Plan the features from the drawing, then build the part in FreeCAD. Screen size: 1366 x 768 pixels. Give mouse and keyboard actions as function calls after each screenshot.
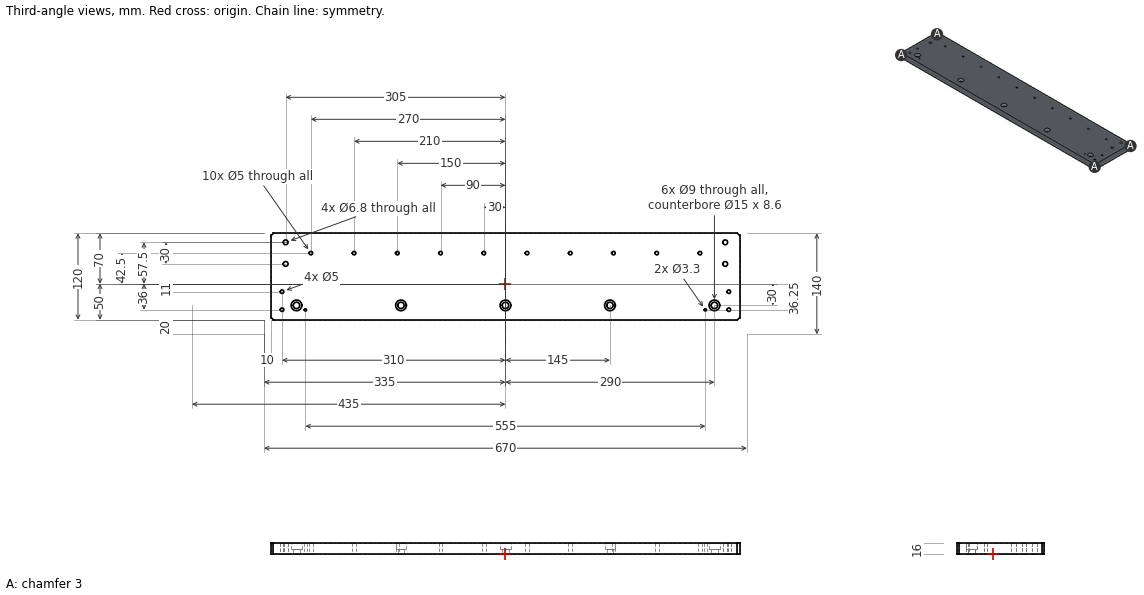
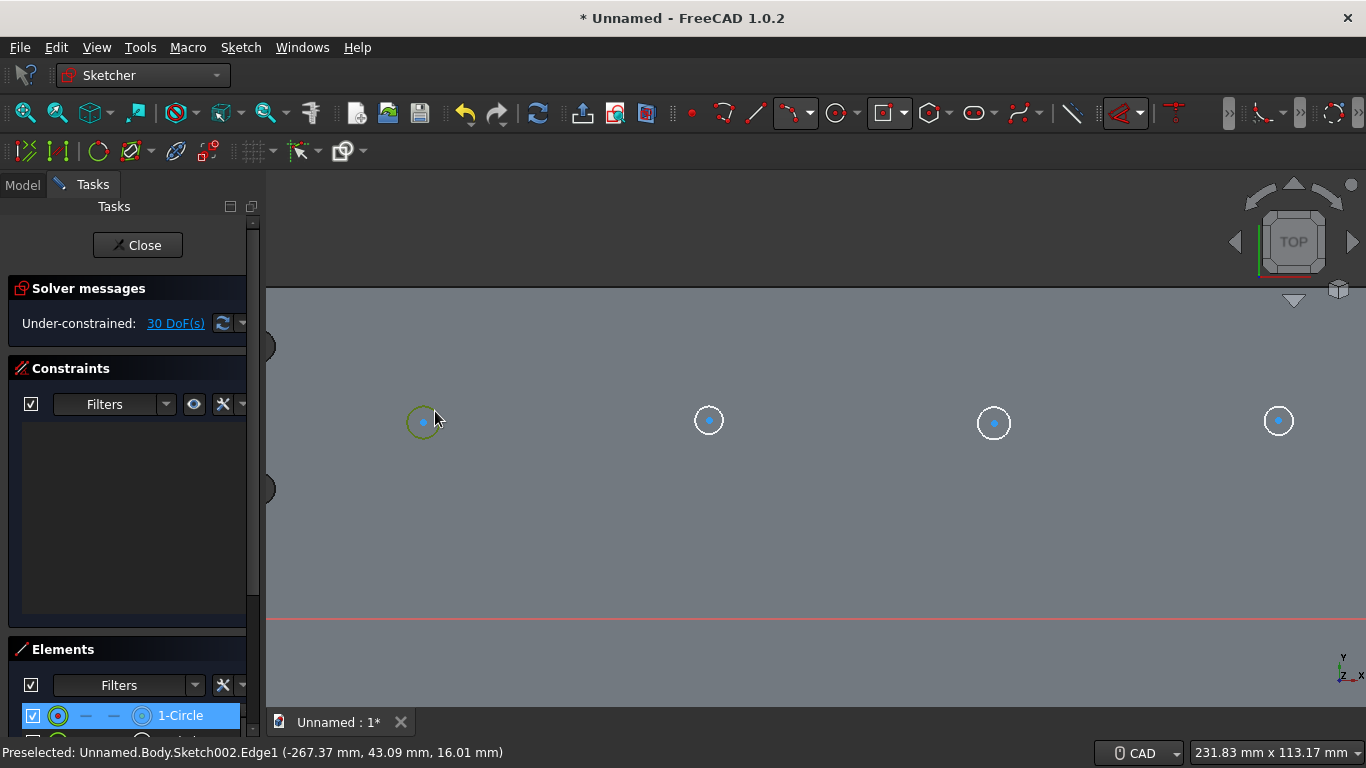
click(719, 410)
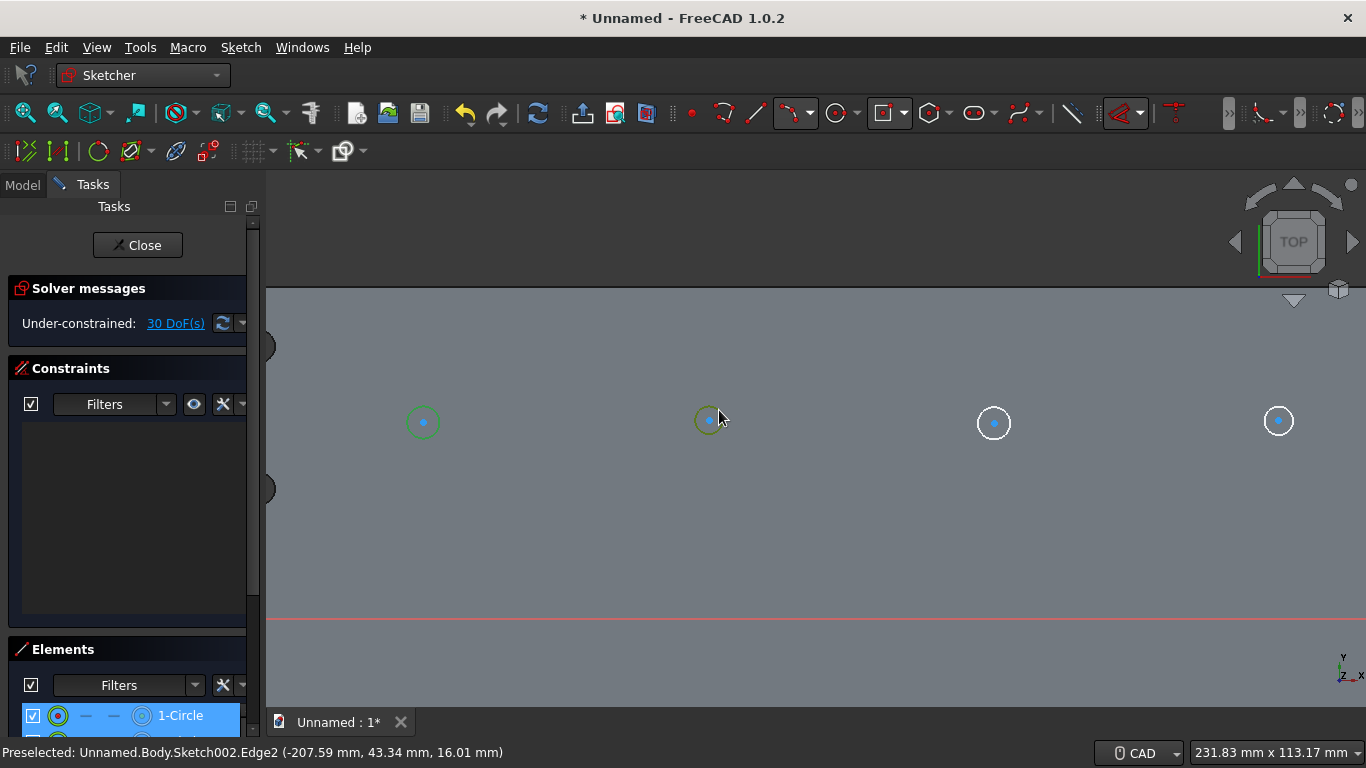
click(1005, 412)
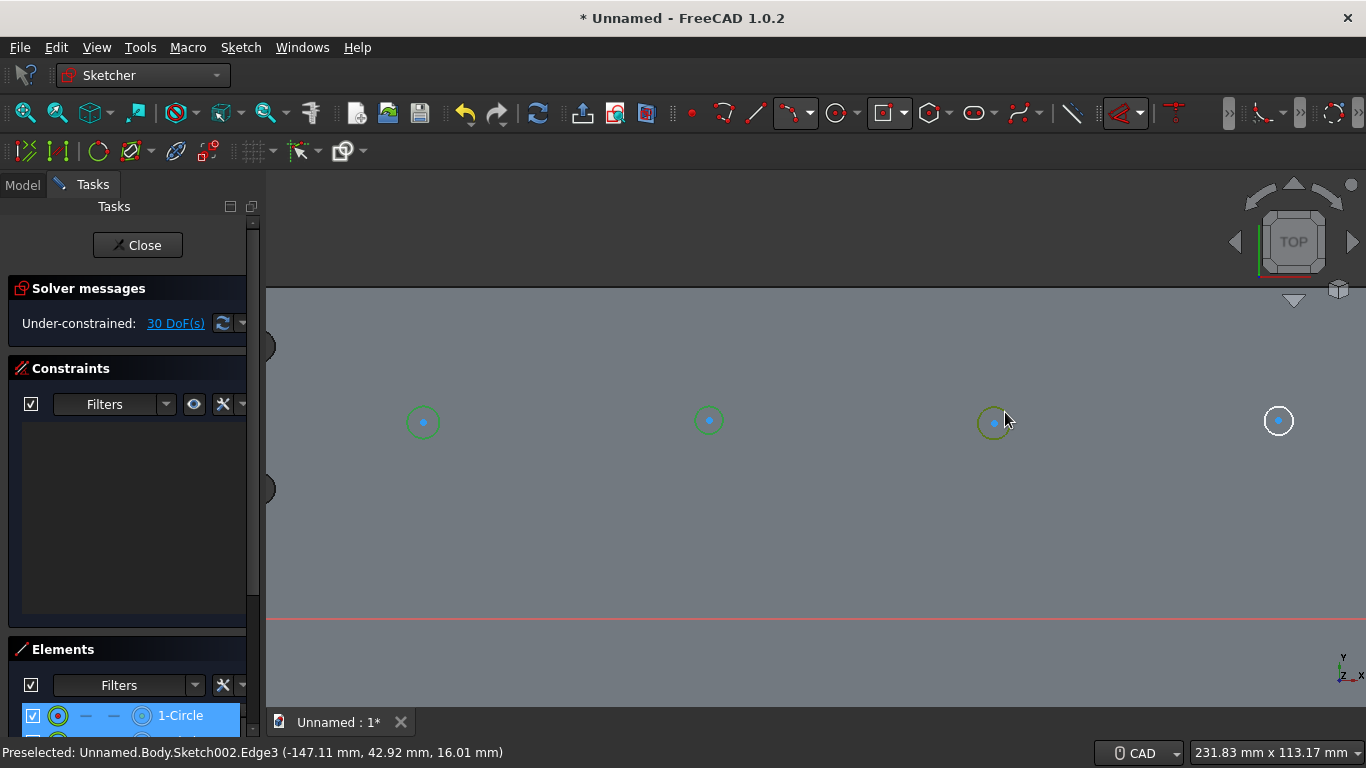
scroll(434, 414, down, 7)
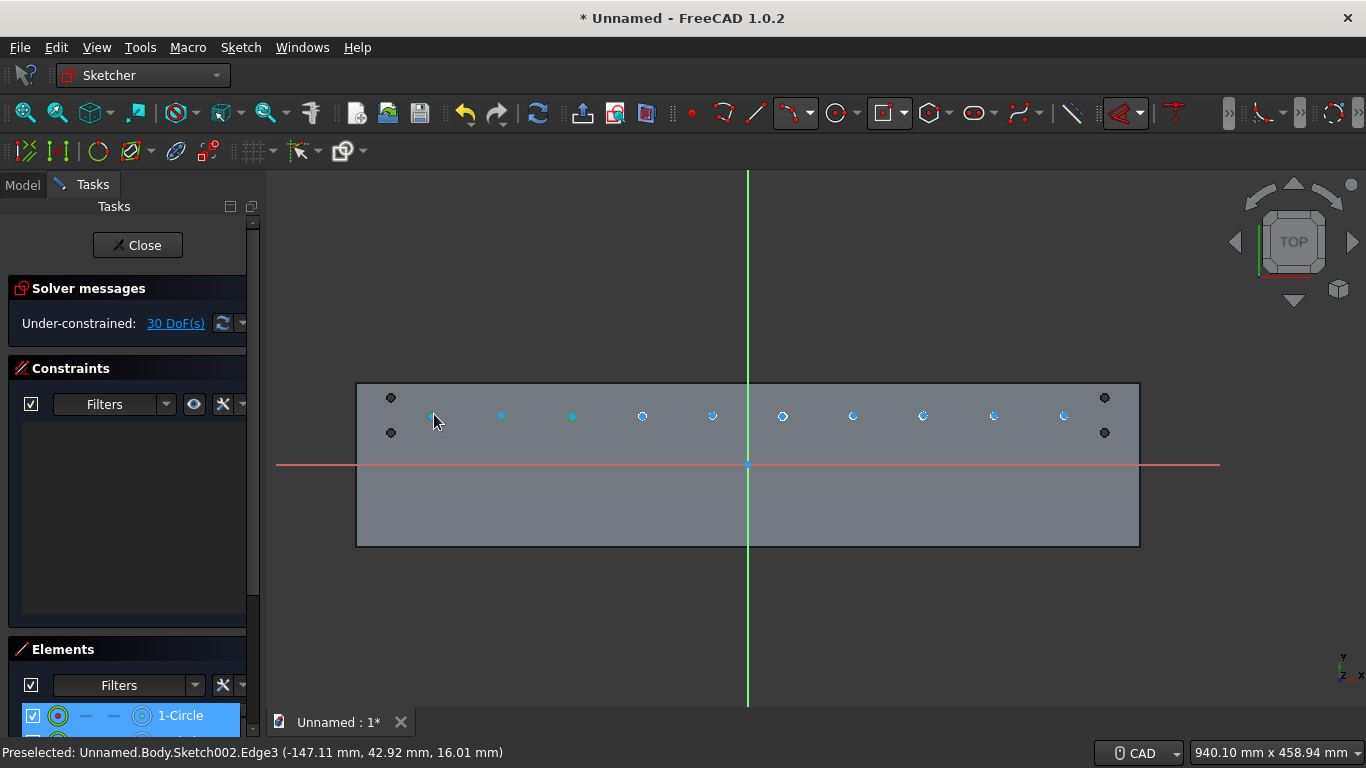
scroll(645, 414, up, 7)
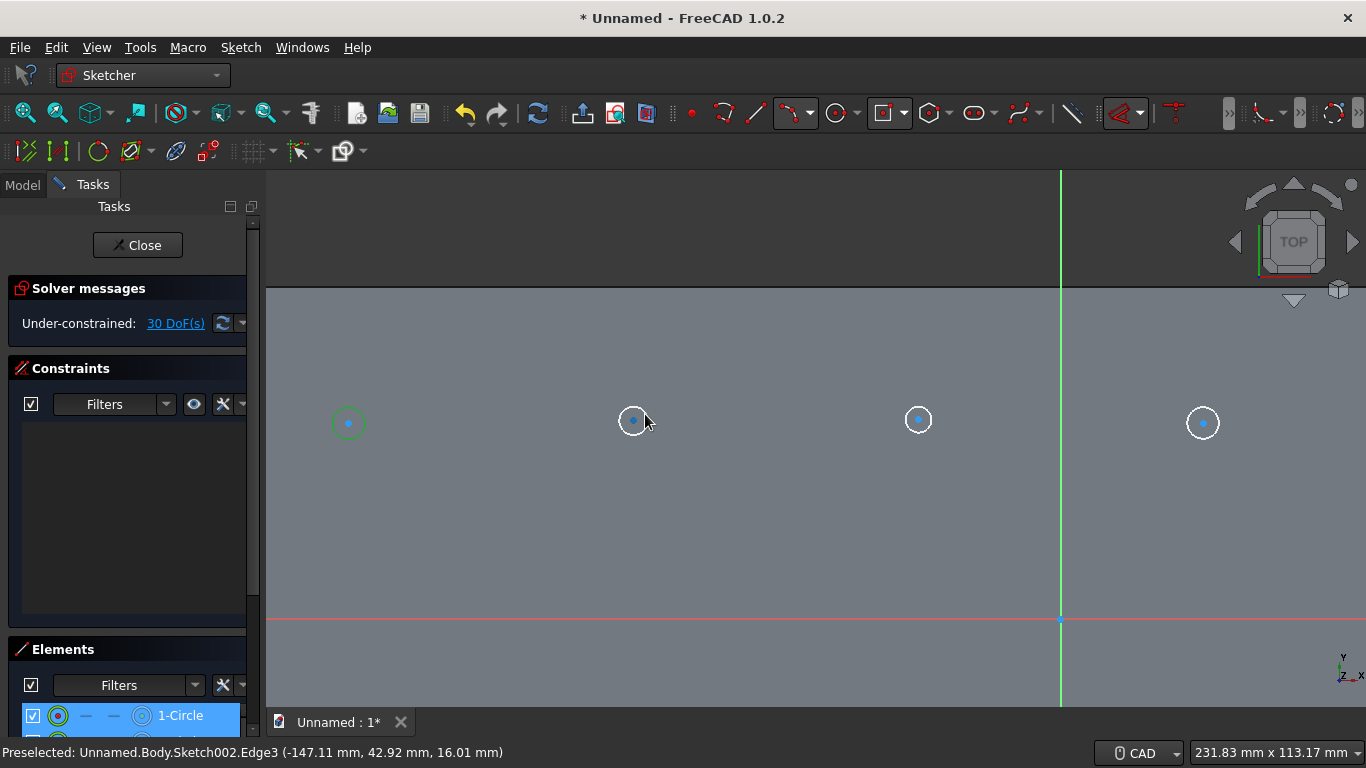
click(644, 411)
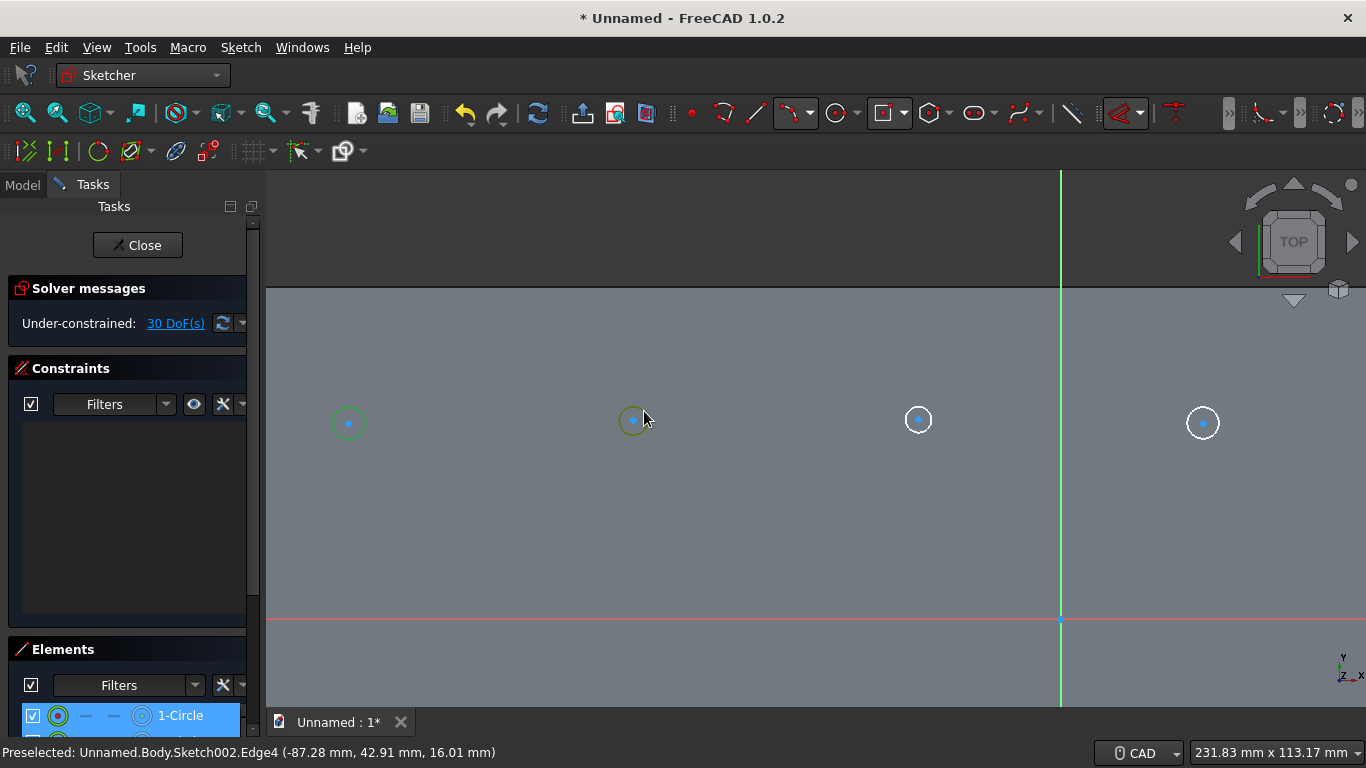
click(928, 411)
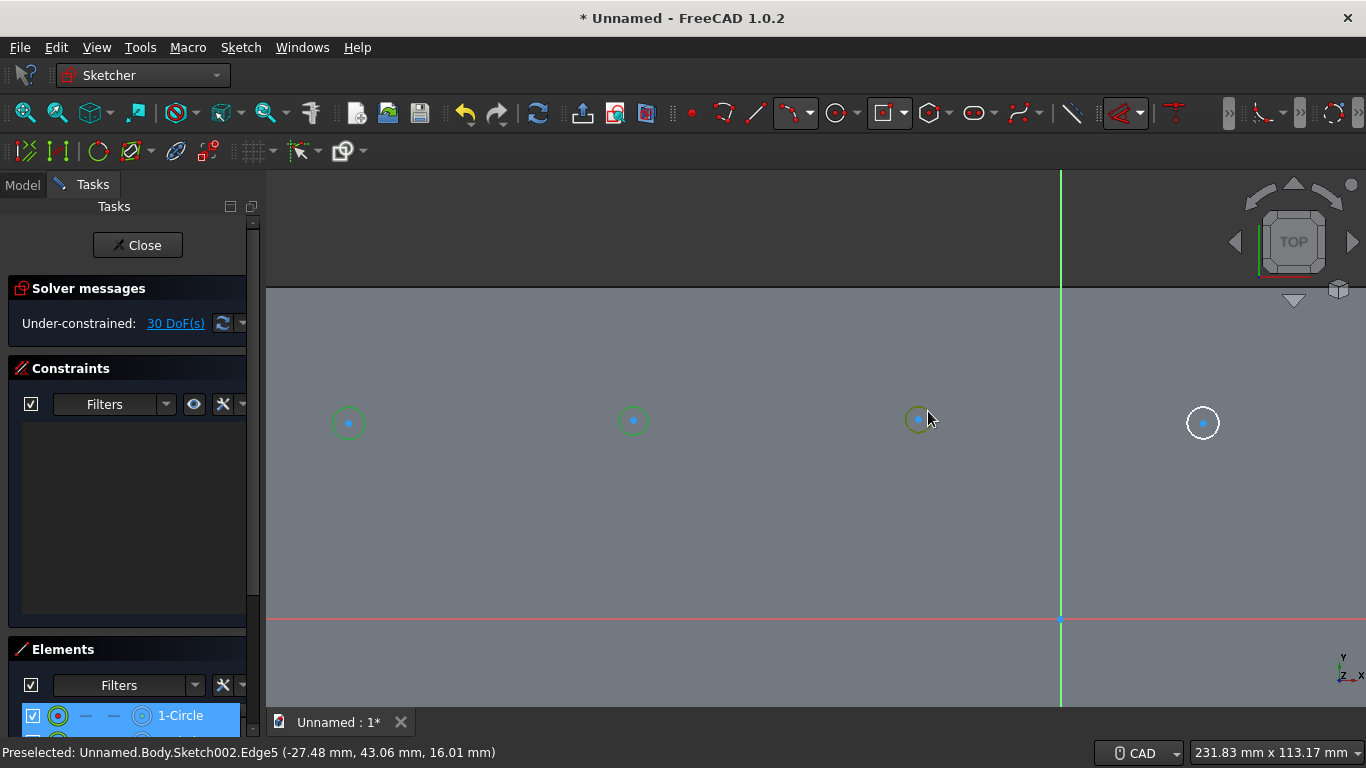
click(1192, 412)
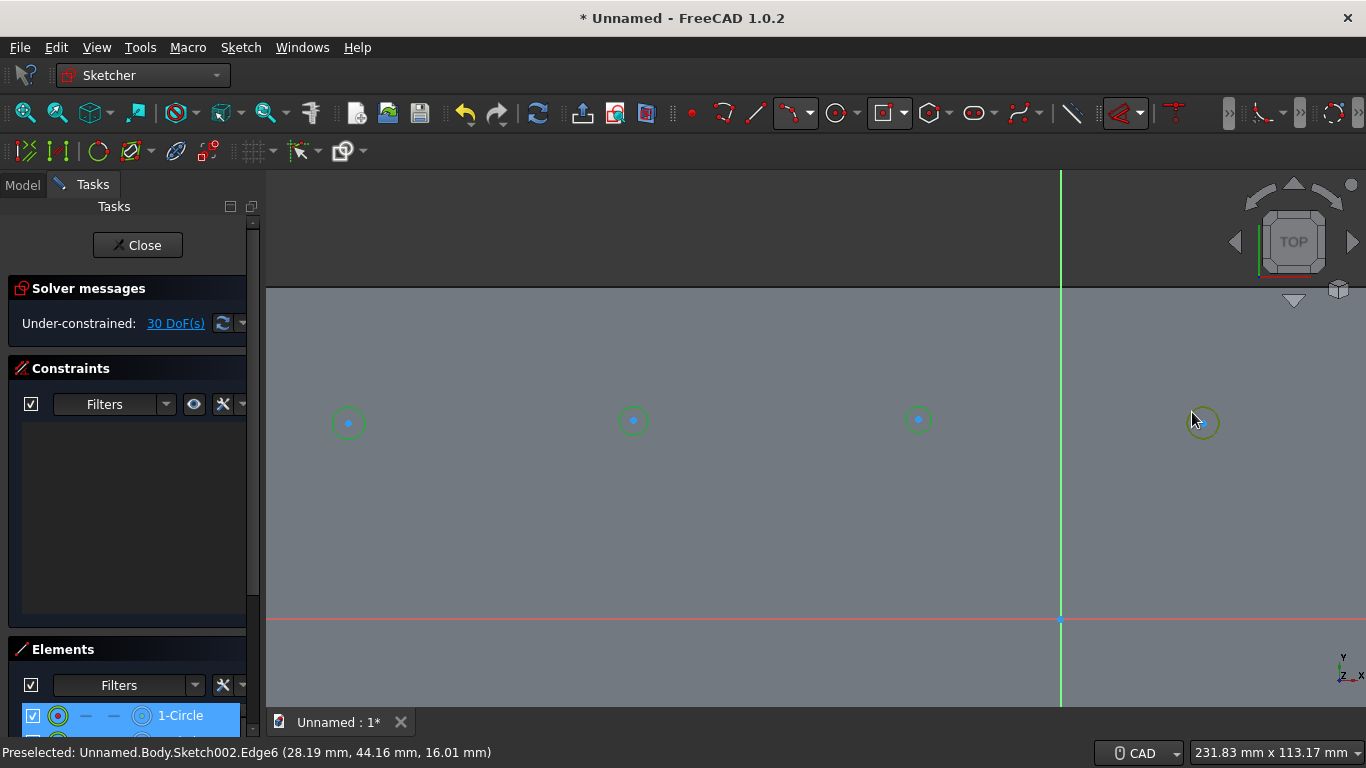
scroll(645, 414, down, 7)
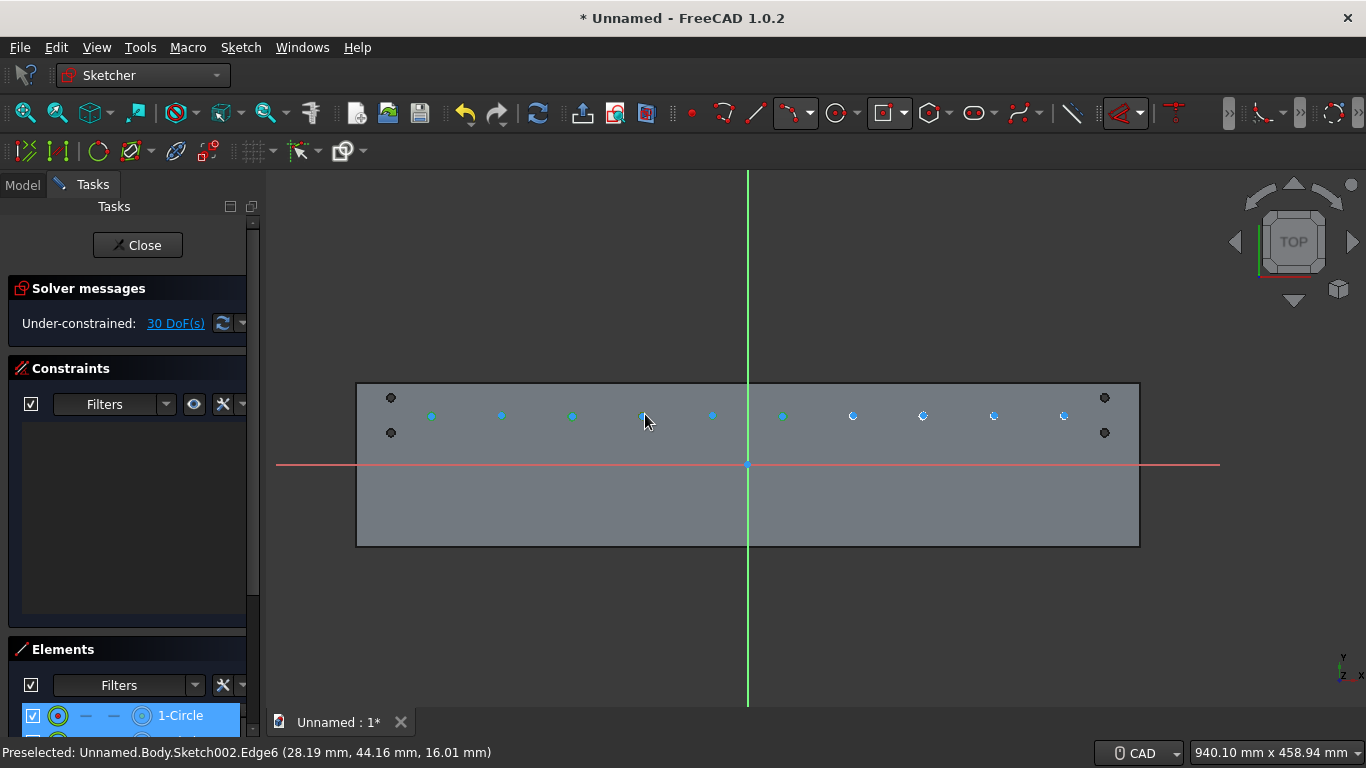
scroll(855, 414, up, 7)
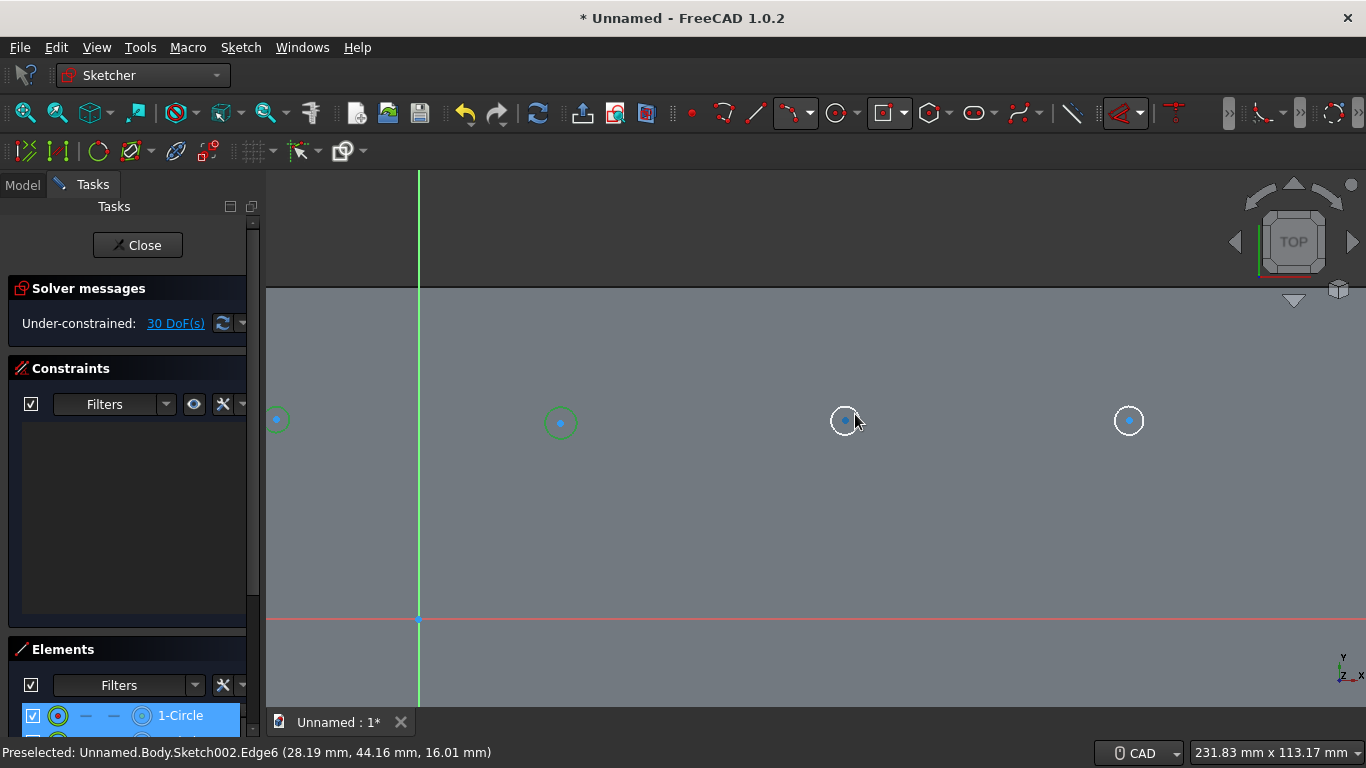
click(855, 411)